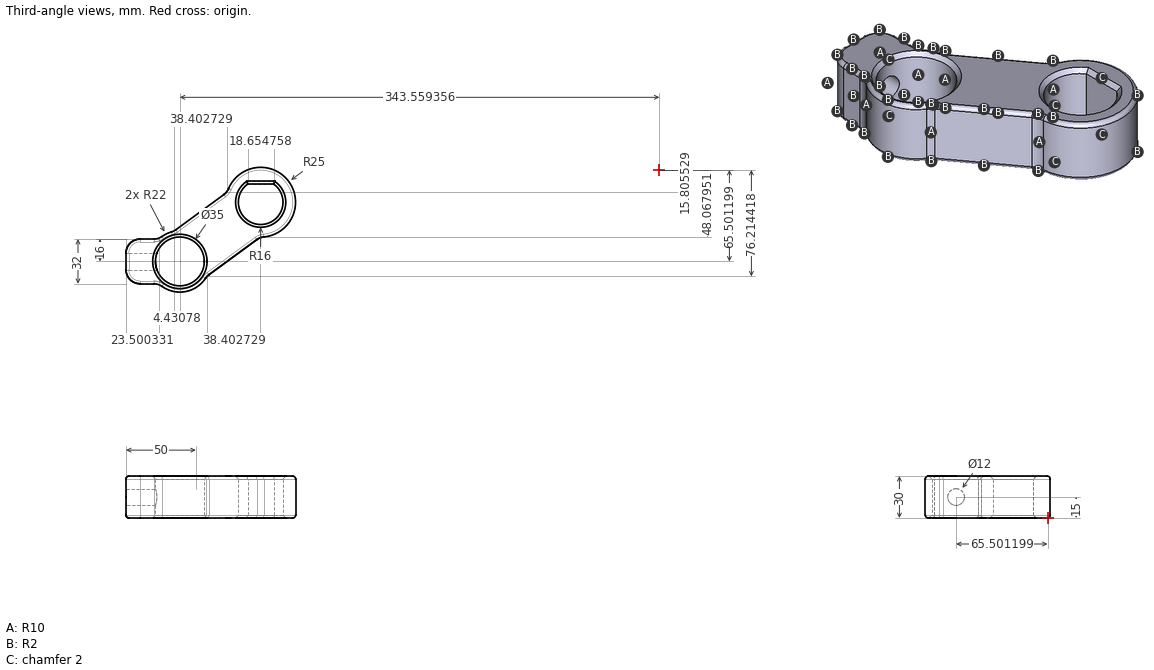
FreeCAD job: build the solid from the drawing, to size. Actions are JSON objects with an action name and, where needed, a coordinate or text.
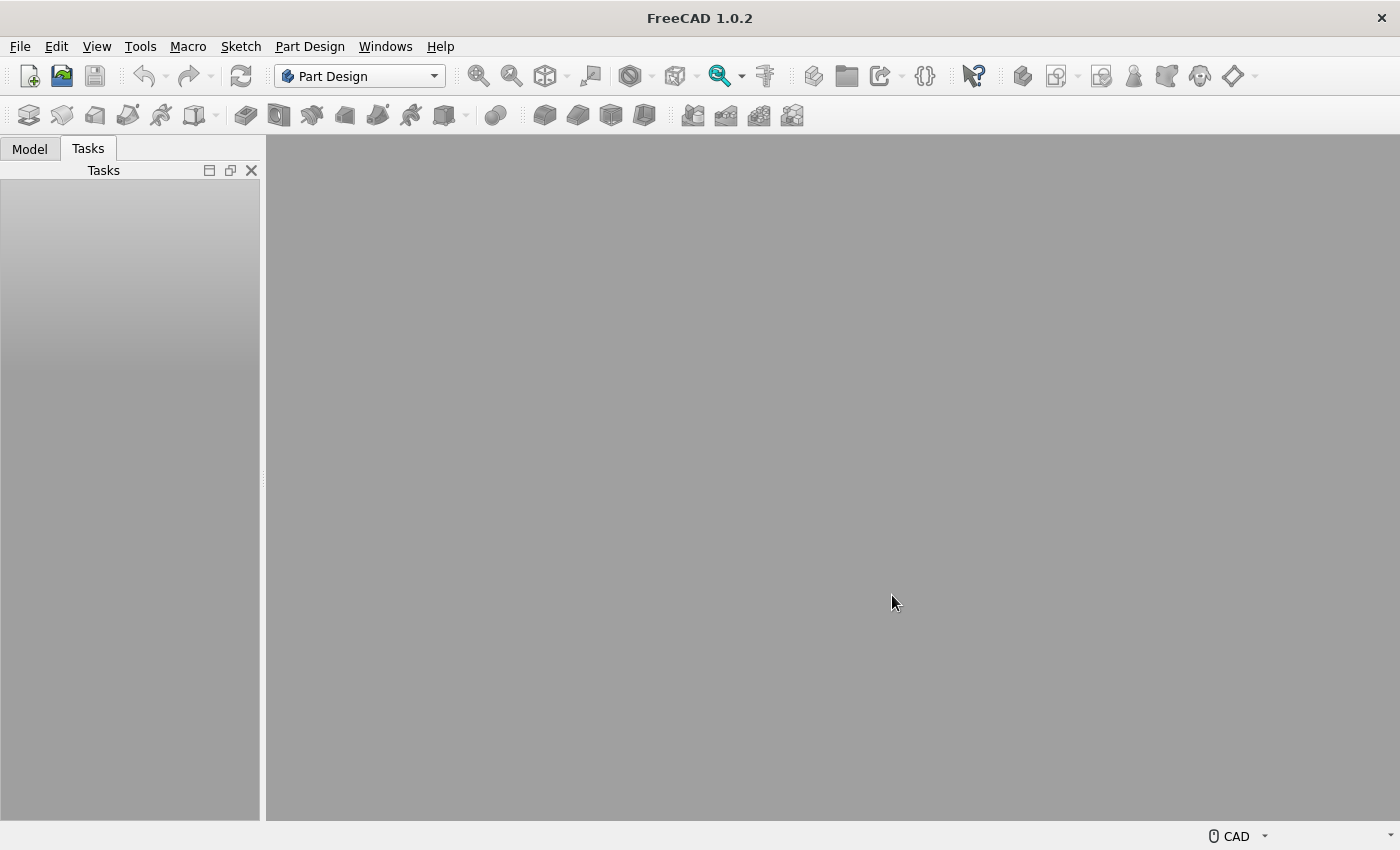
{"action": "left_click", "coordinate": [29, 76]}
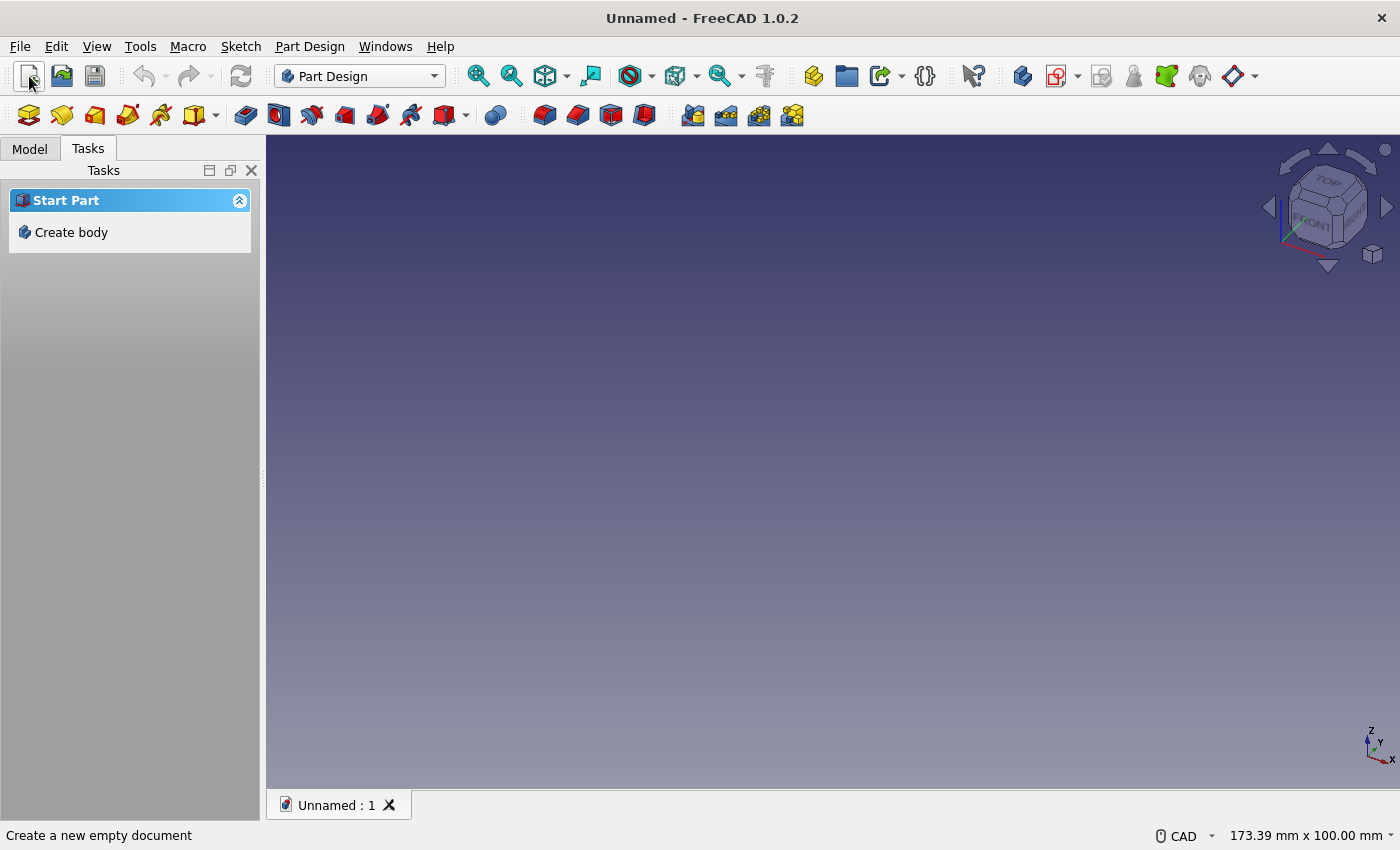
{"action": "left_click", "coordinate": [1056, 76]}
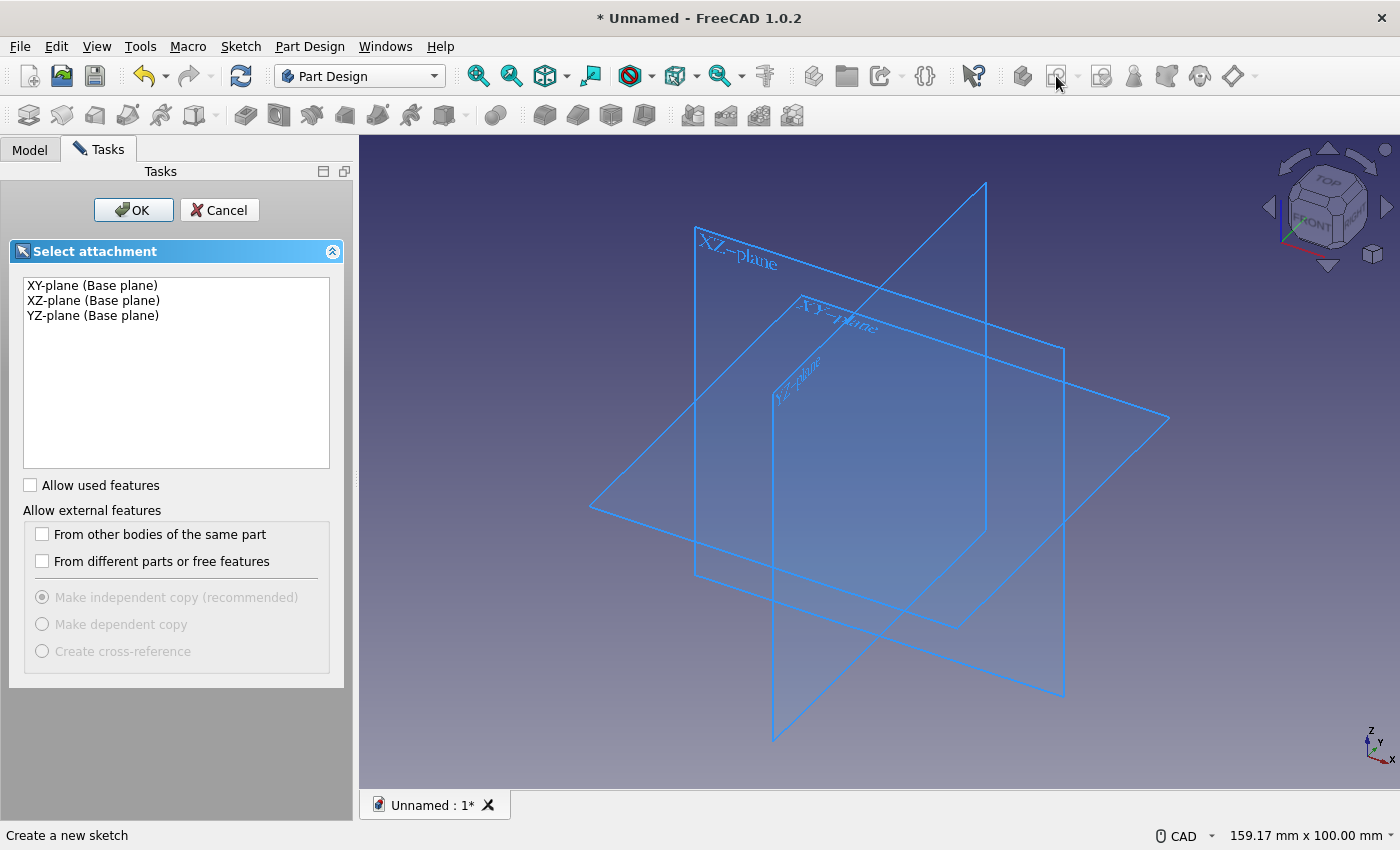
{"action": "left_click", "coordinate": [84, 286]}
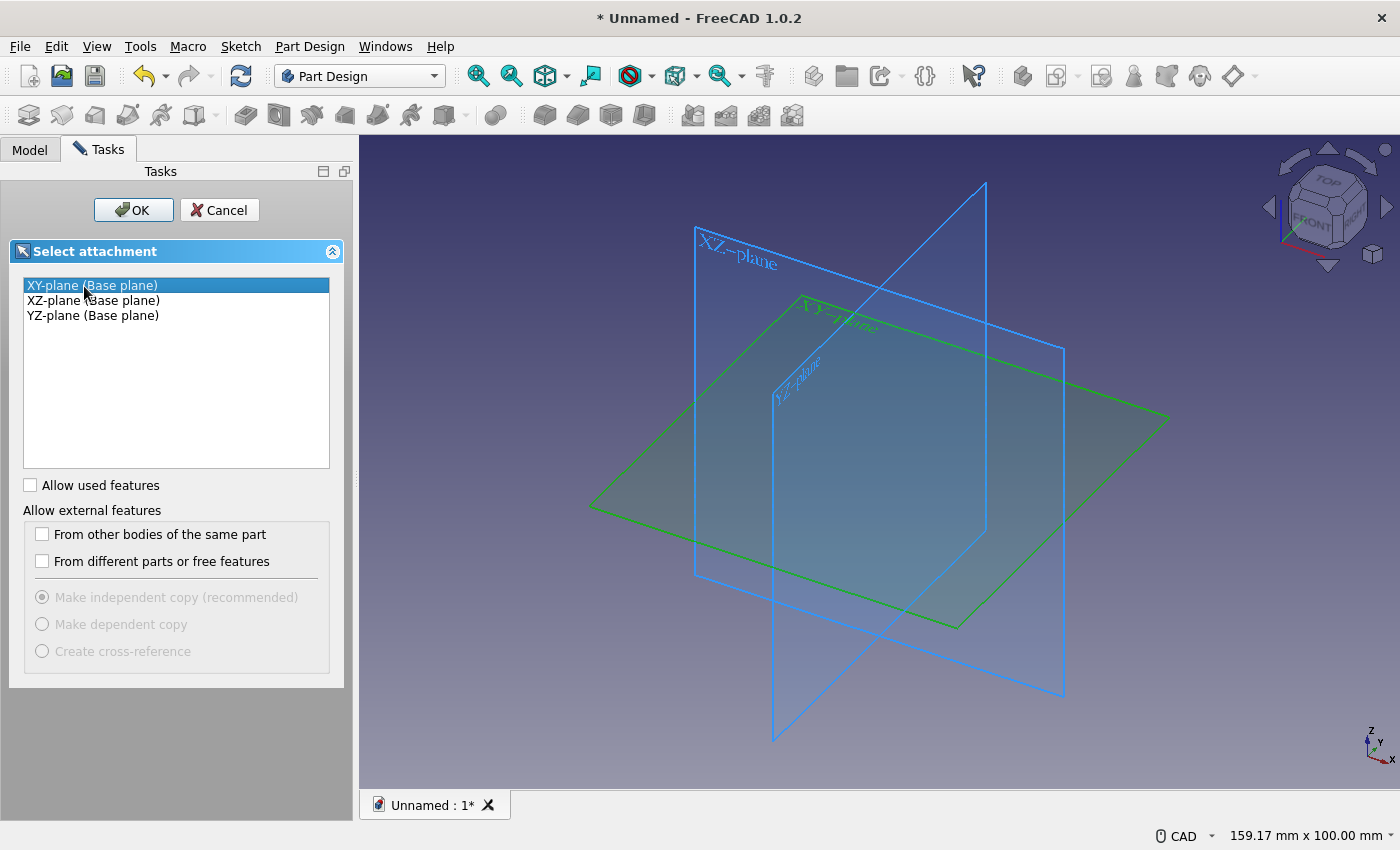
{"action": "left_click", "coordinate": [134, 210]}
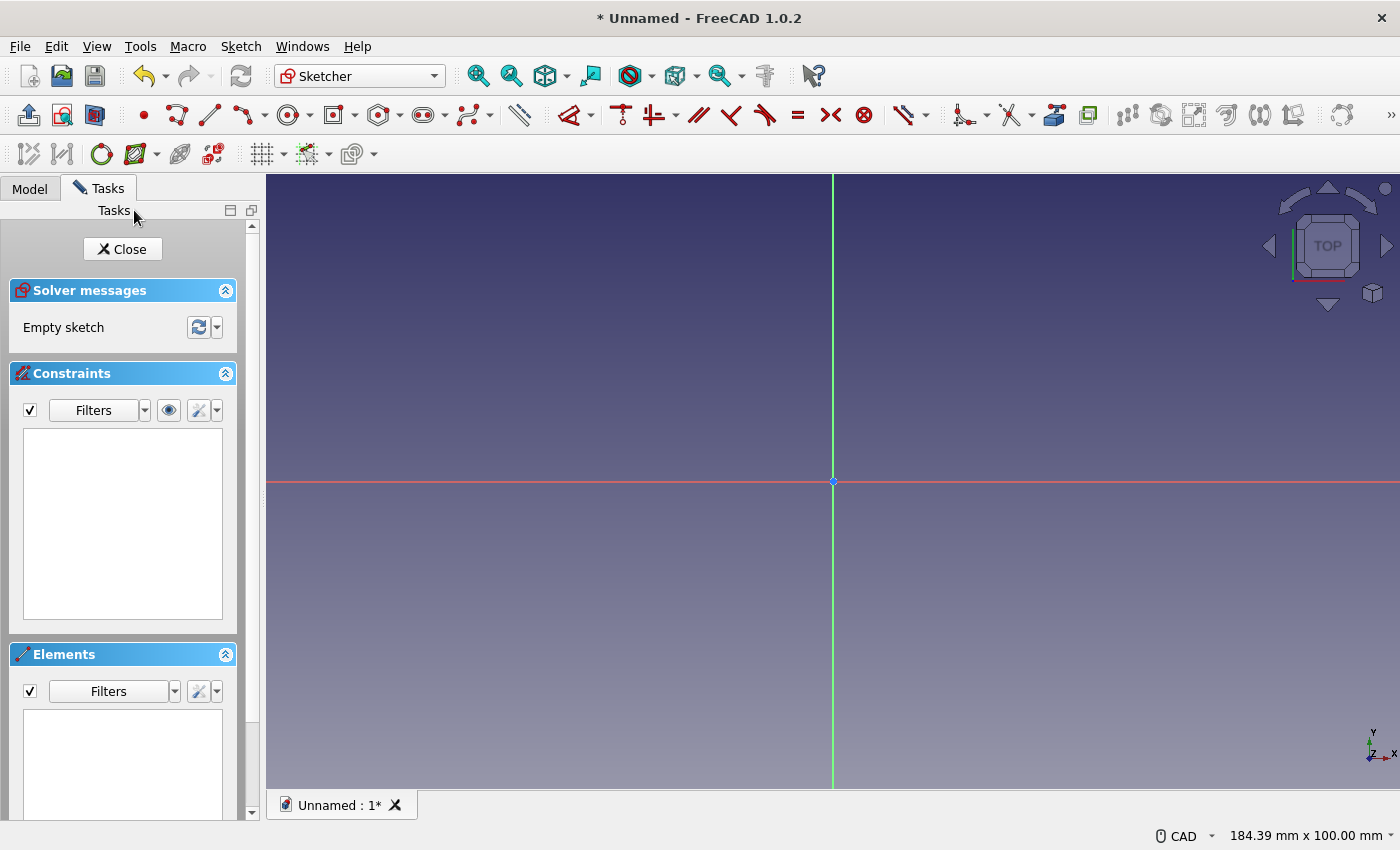
{"action": "scroll", "coordinate": [764, 482], "scroll_direction": "down", "scroll_amount": 5}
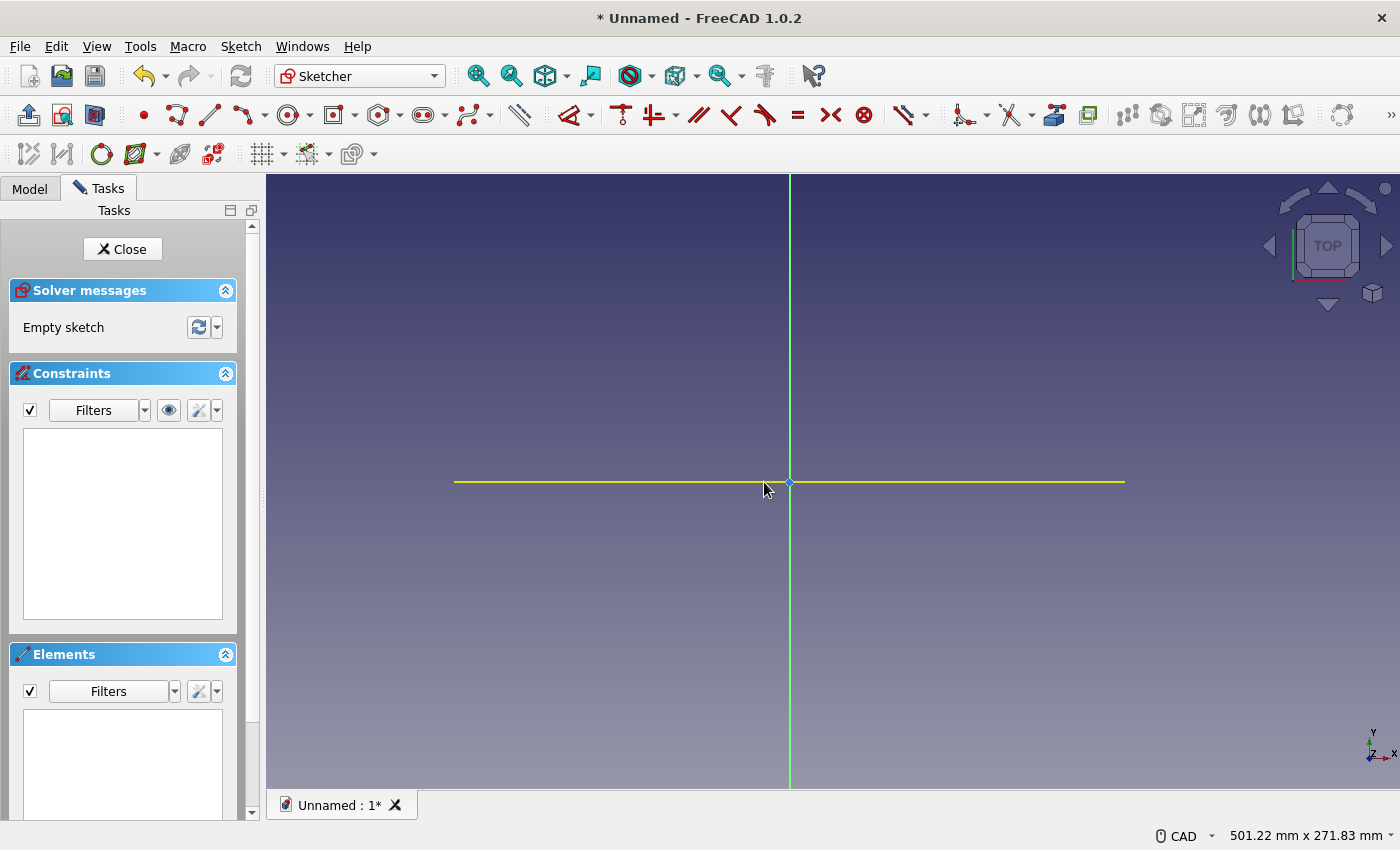
{"action": "scroll", "coordinate": [764, 482], "scroll_direction": "down", "scroll_amount": 5}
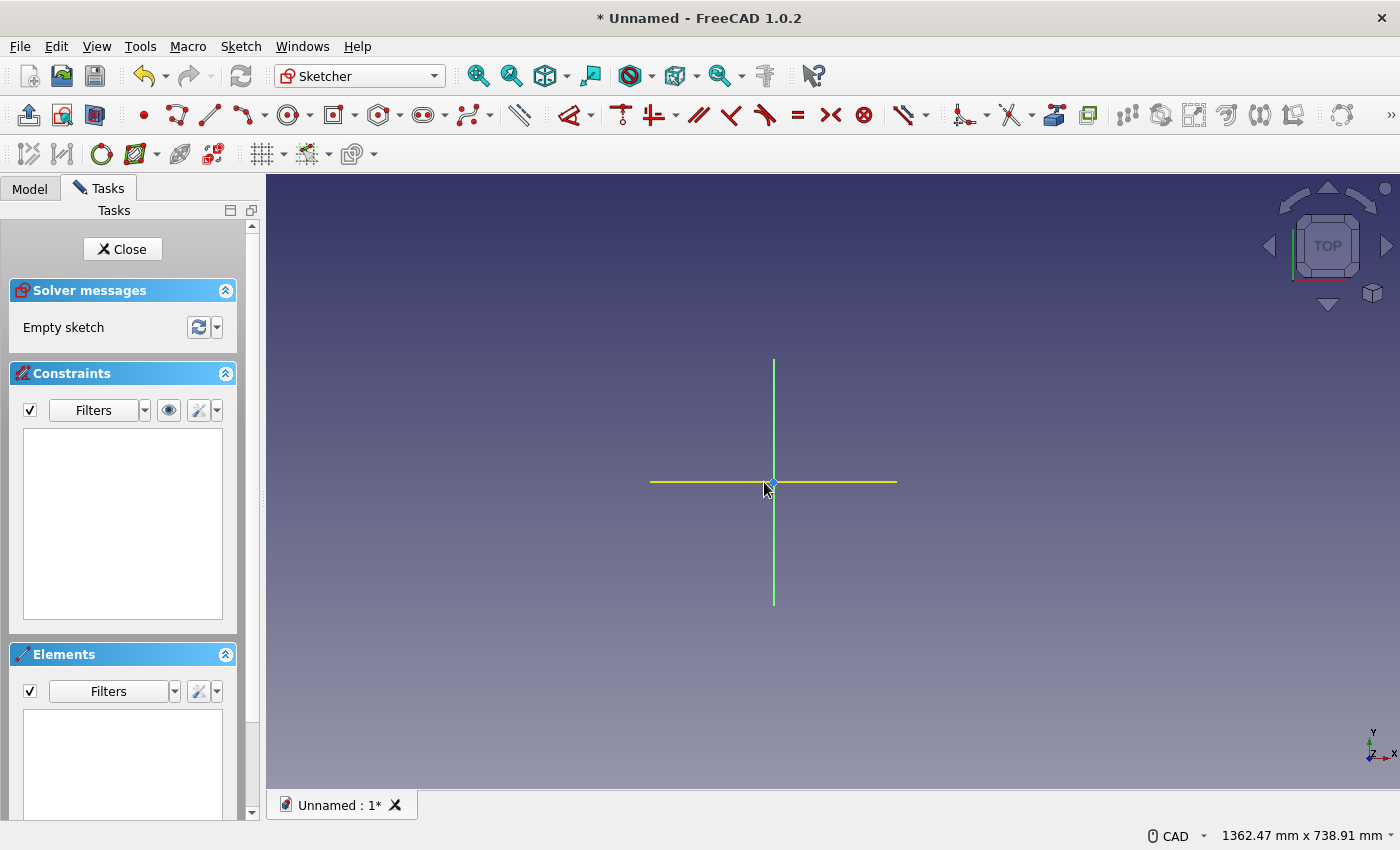
{"action": "scroll", "coordinate": [453, 530], "scroll_direction": "up", "scroll_amount": 9}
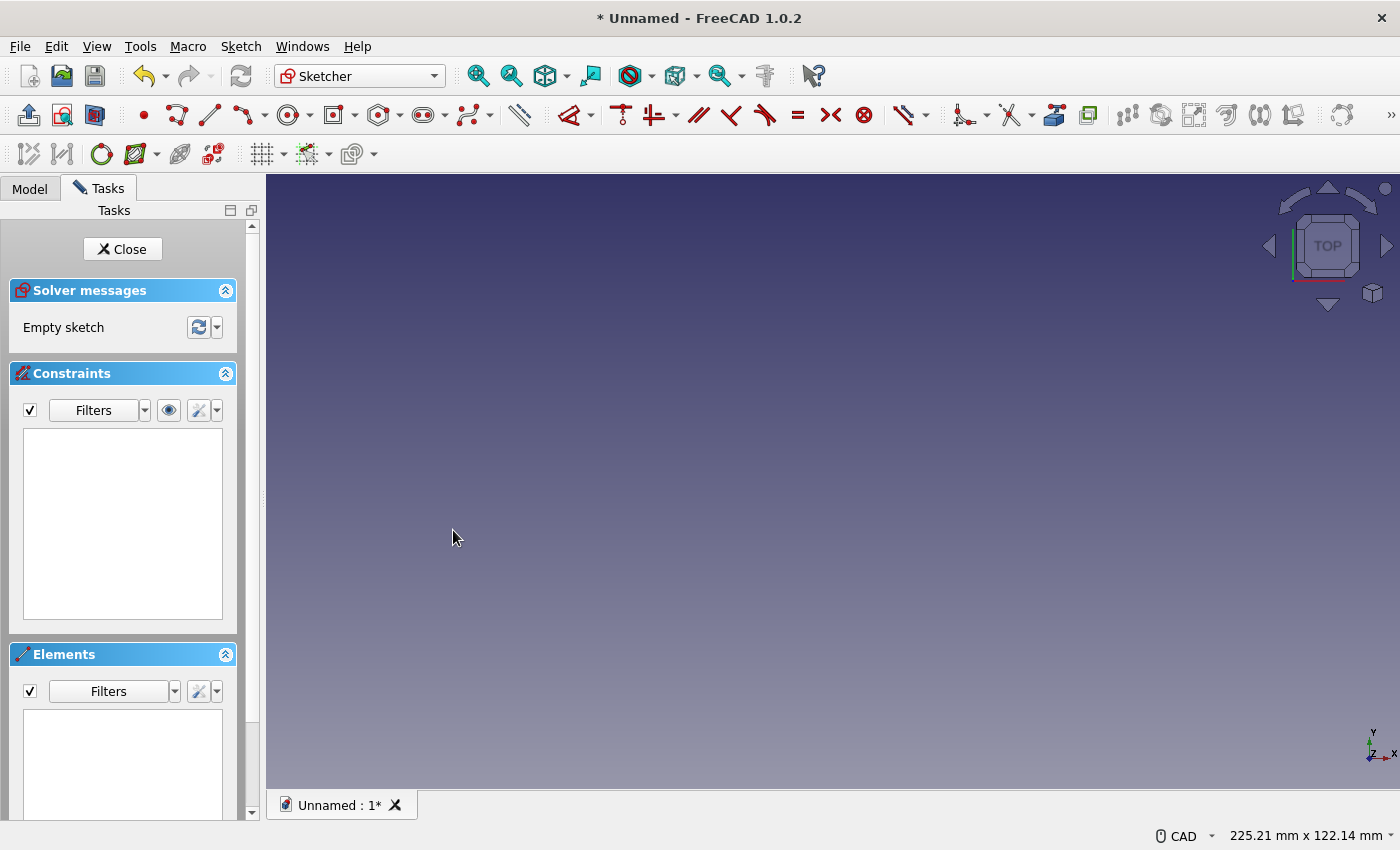
{"action": "left_click", "coordinate": [210, 116]}